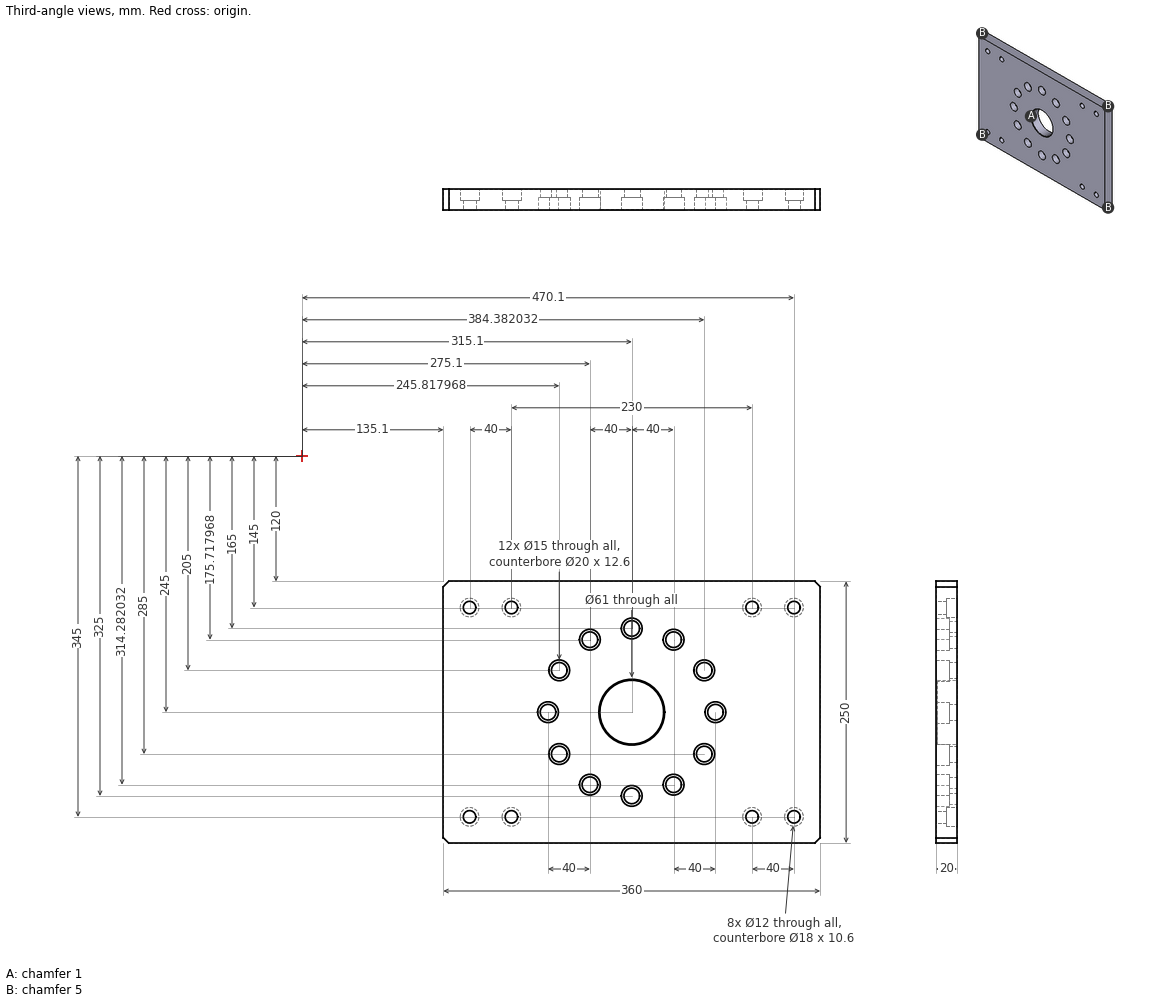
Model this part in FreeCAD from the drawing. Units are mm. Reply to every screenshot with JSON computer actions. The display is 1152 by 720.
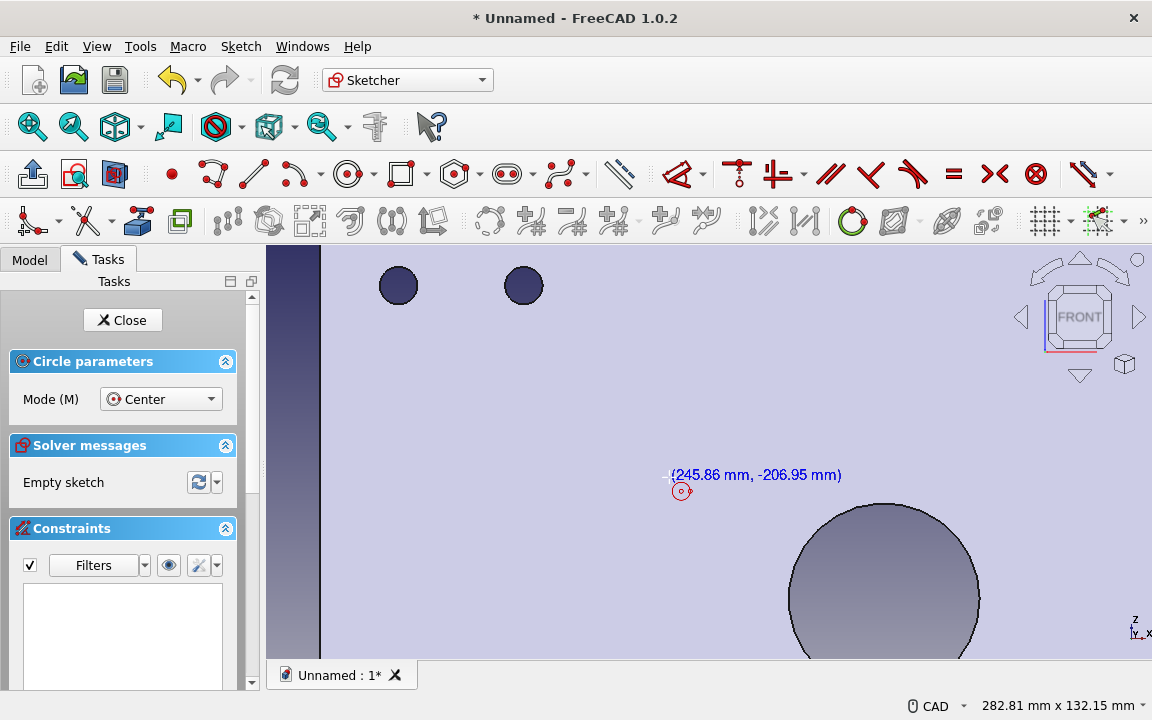
{"action": "scroll", "coordinate": [677, 485], "scroll_direction": "down", "scroll_amount": 7}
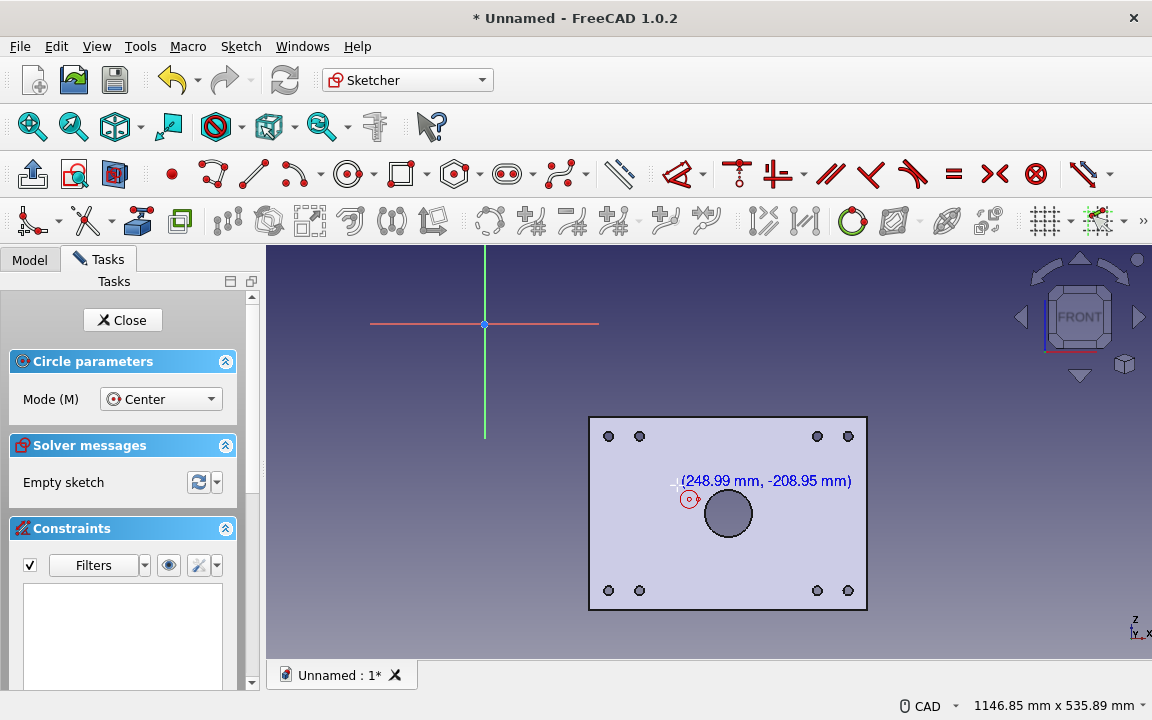
{"action": "left_click", "coordinate": [675, 483]}
{"action": "mouse_move", "coordinate": [679, 479]}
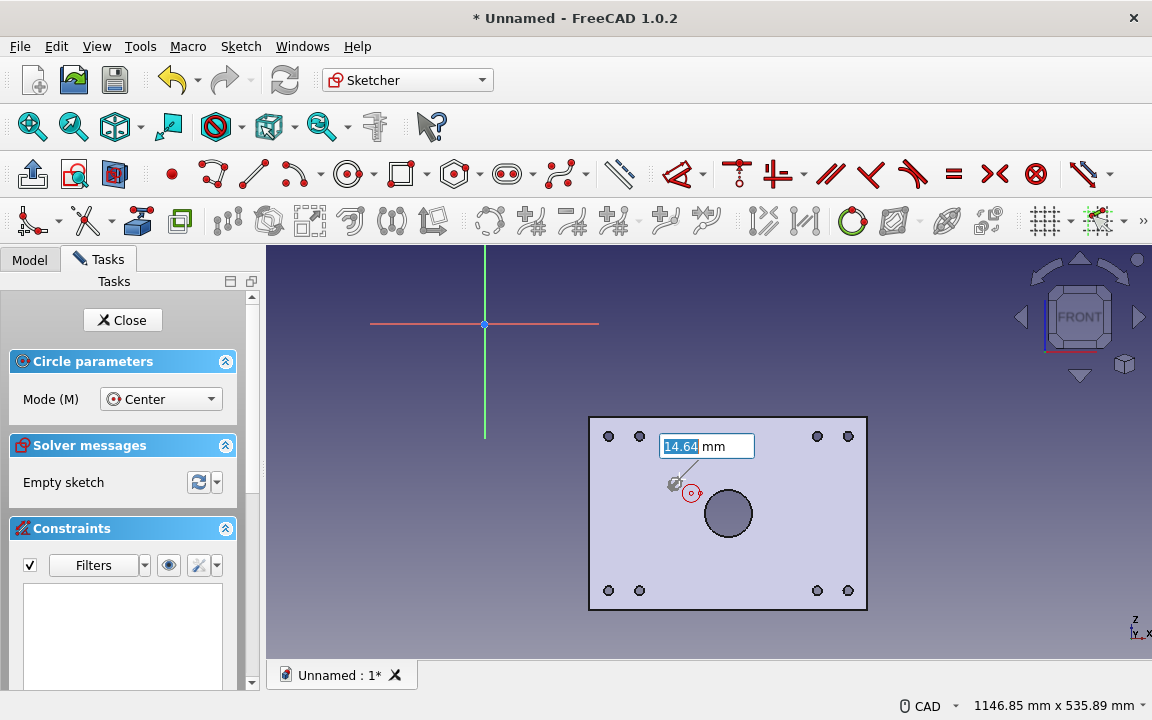
{"action": "type", "text": "15"}
{"action": "key", "text": "Return"}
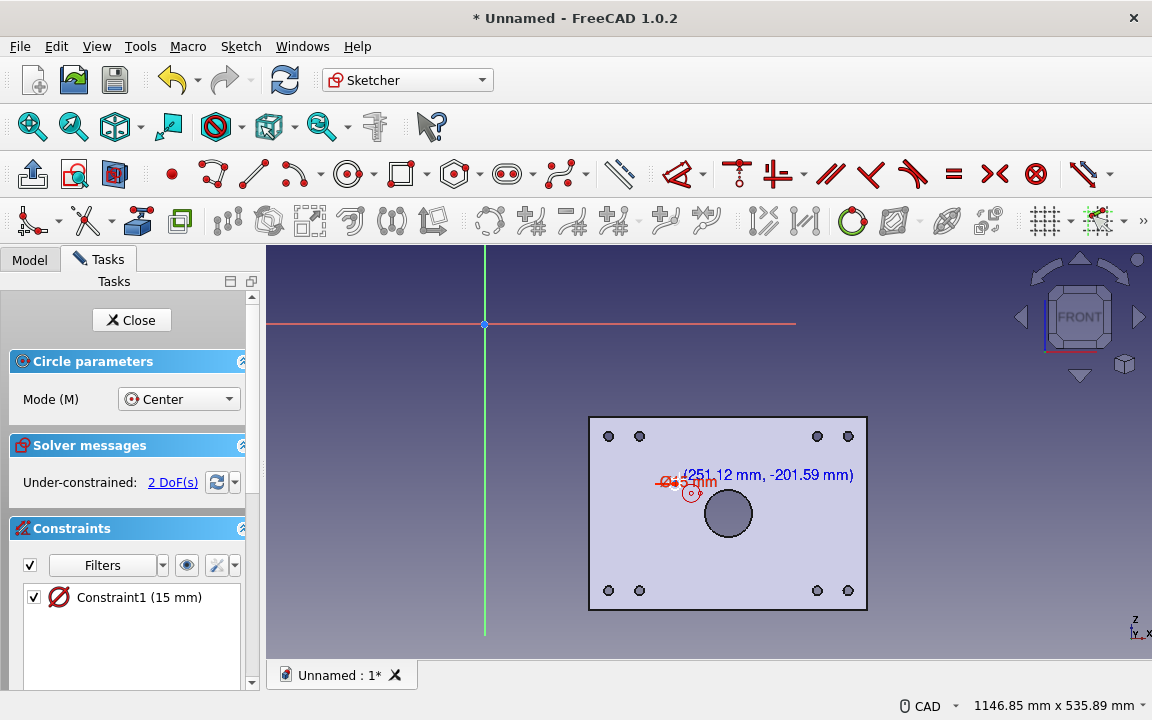
{"action": "scroll", "coordinate": [698, 460], "scroll_direction": "up", "scroll_amount": 7}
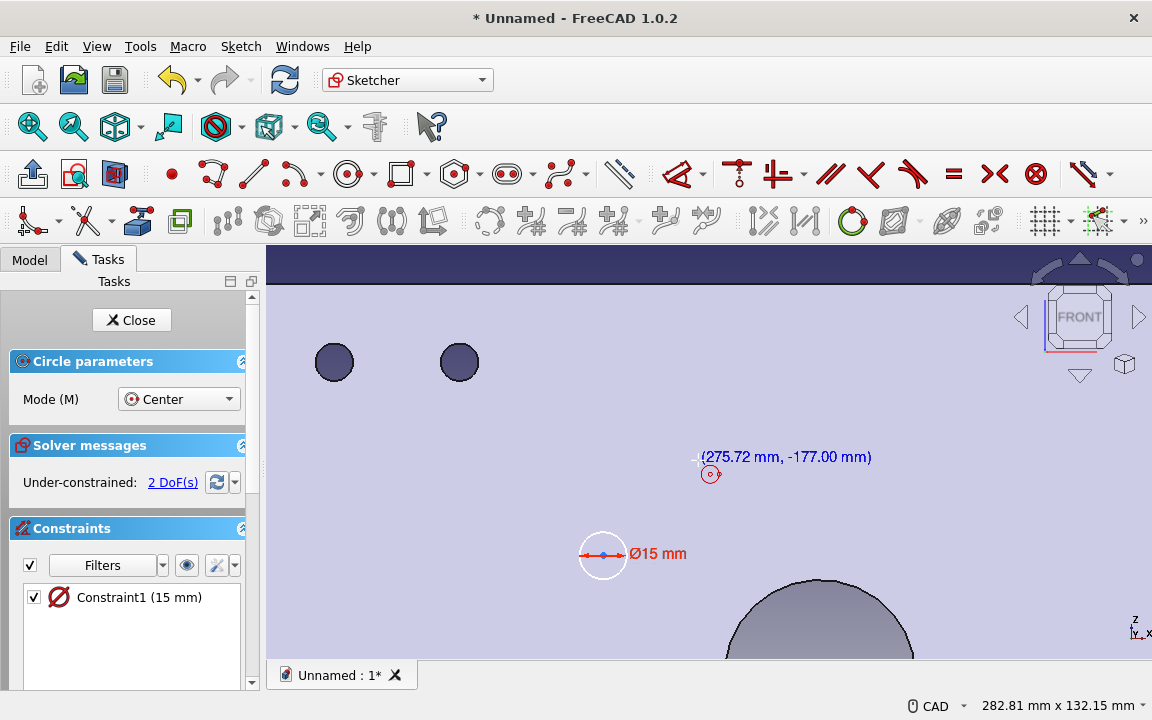
{"action": "scroll", "coordinate": [698, 460], "scroll_direction": "down", "scroll_amount": 7}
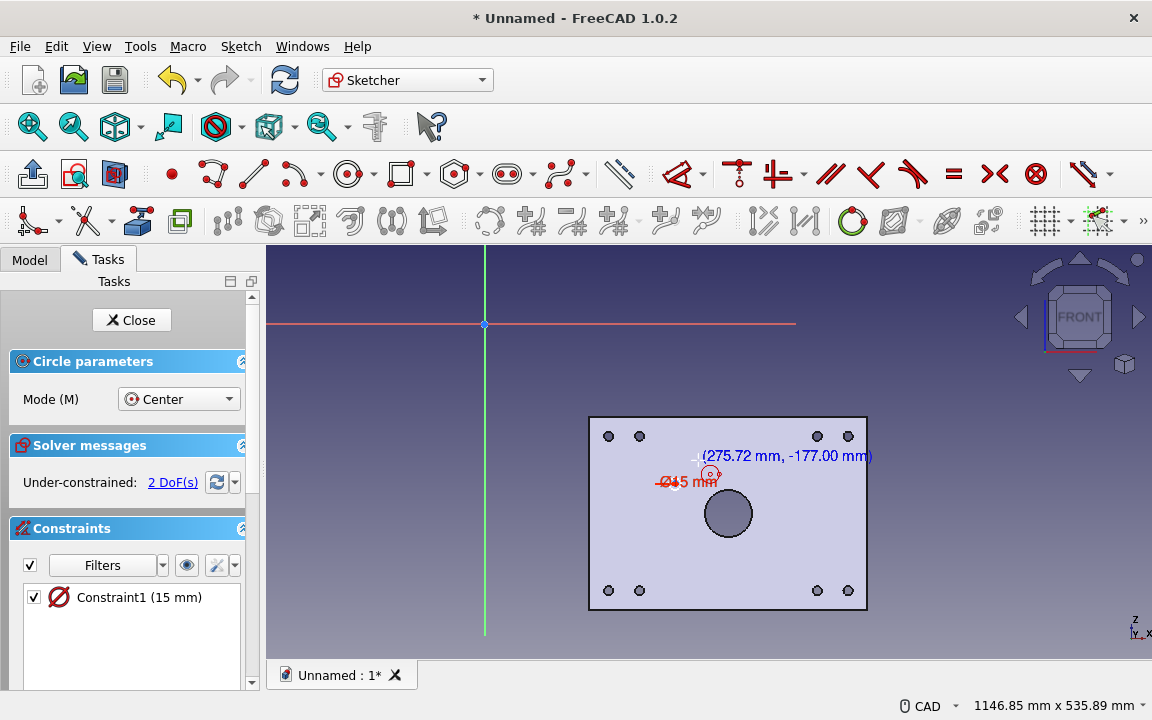
{"action": "left_click", "coordinate": [698, 460]}
{"action": "mouse_move", "coordinate": [702, 456]}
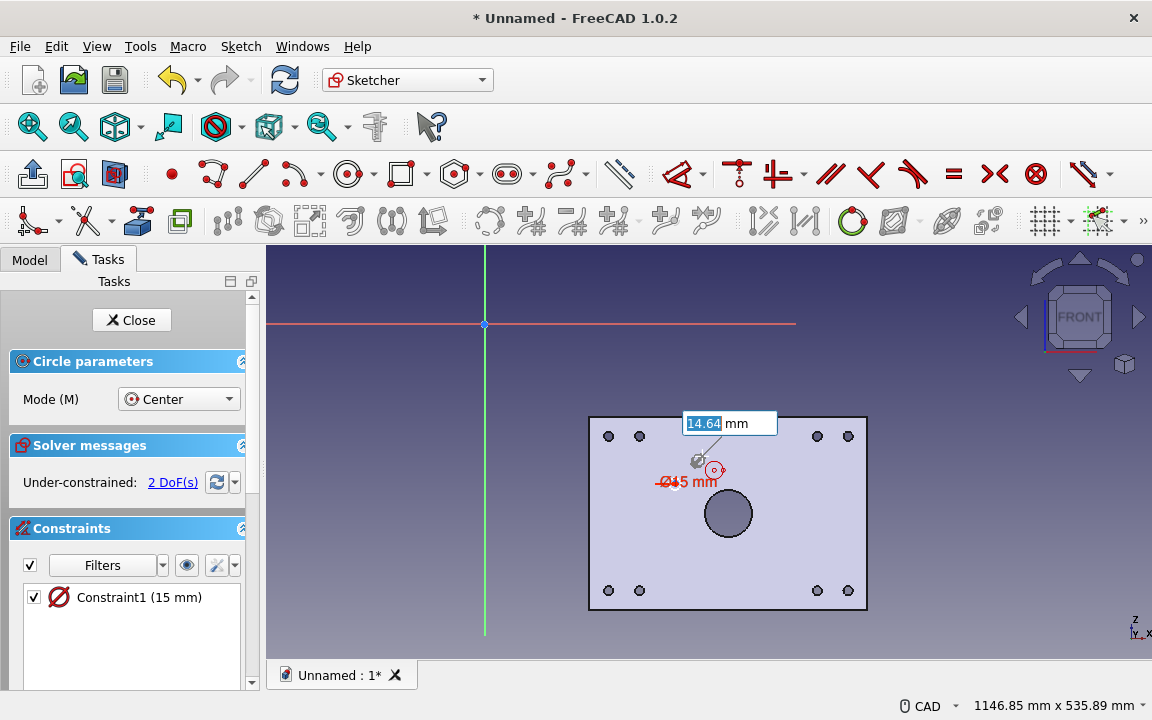
{"action": "type", "text": "15"}
{"action": "key", "text": "Return"}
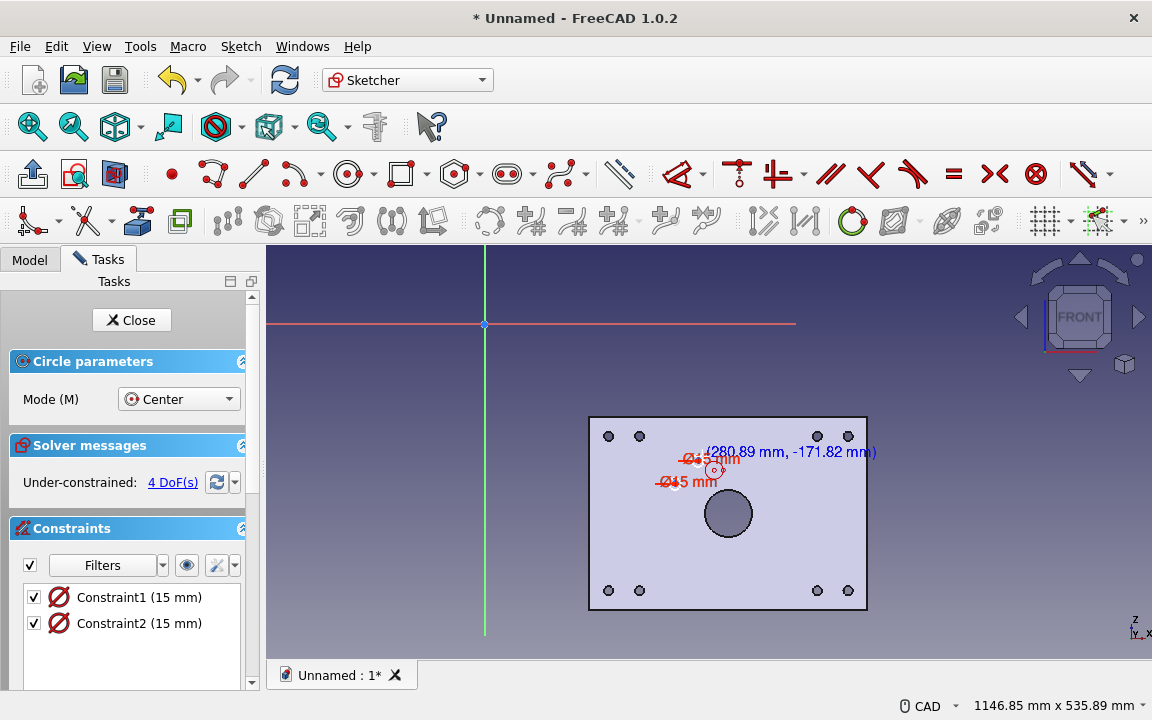
{"action": "scroll", "coordinate": [728, 452], "scroll_direction": "up", "scroll_amount": 7}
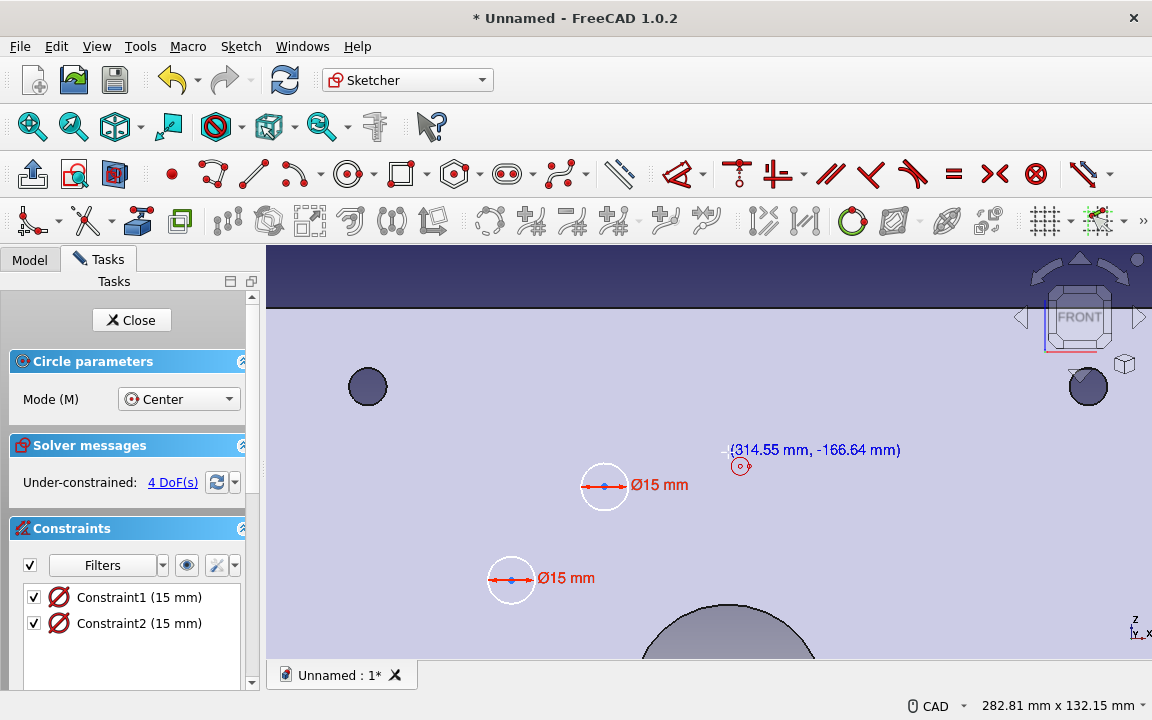
{"action": "scroll", "coordinate": [729, 452], "scroll_direction": "down", "scroll_amount": 7}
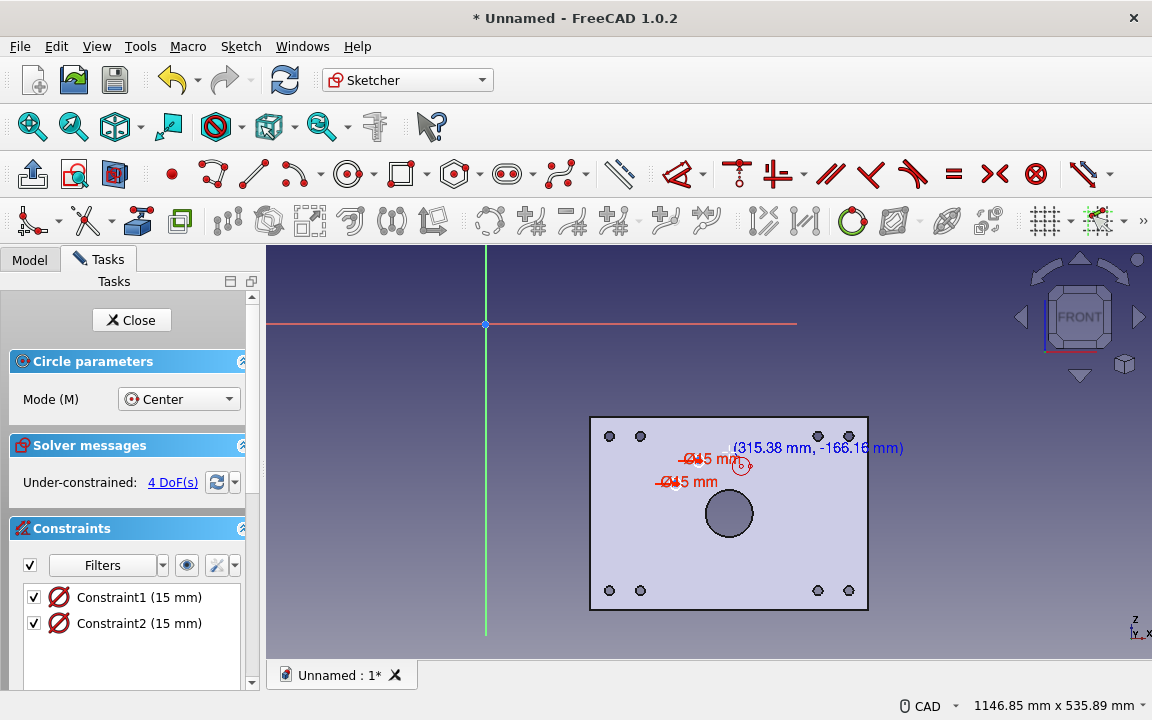
{"action": "left_click", "coordinate": [729, 452]}
{"action": "mouse_move", "coordinate": [733, 448]}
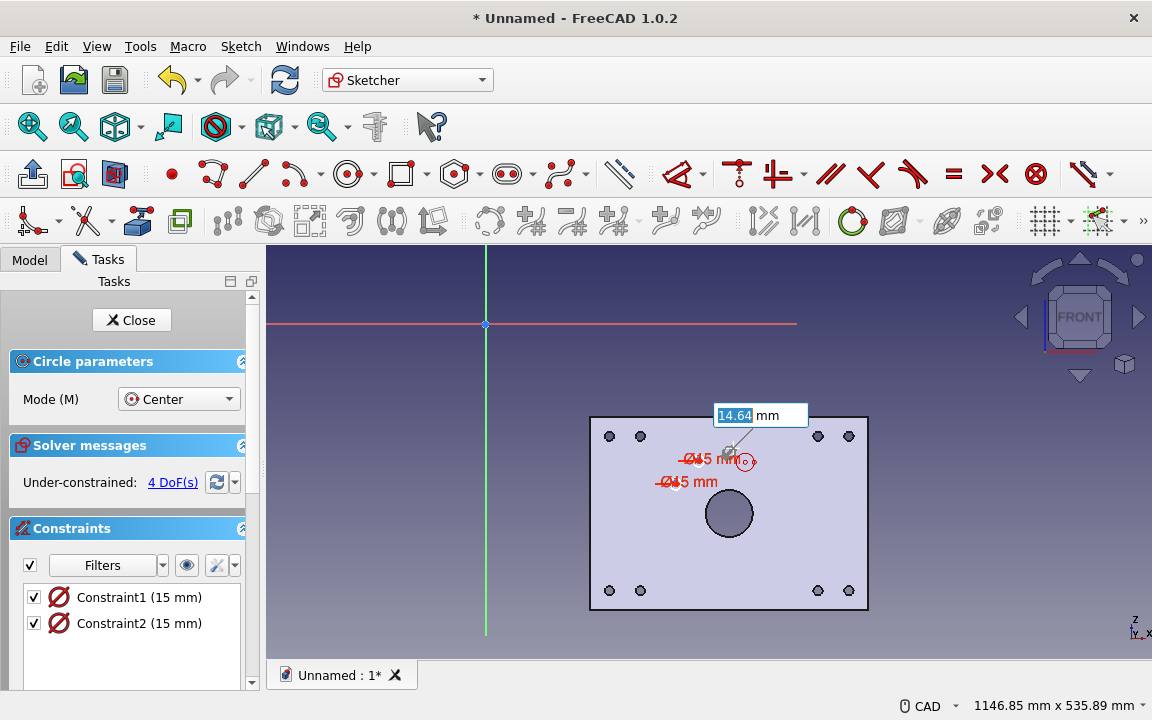
{"action": "type", "text": "15"}
{"action": "key", "text": "Return"}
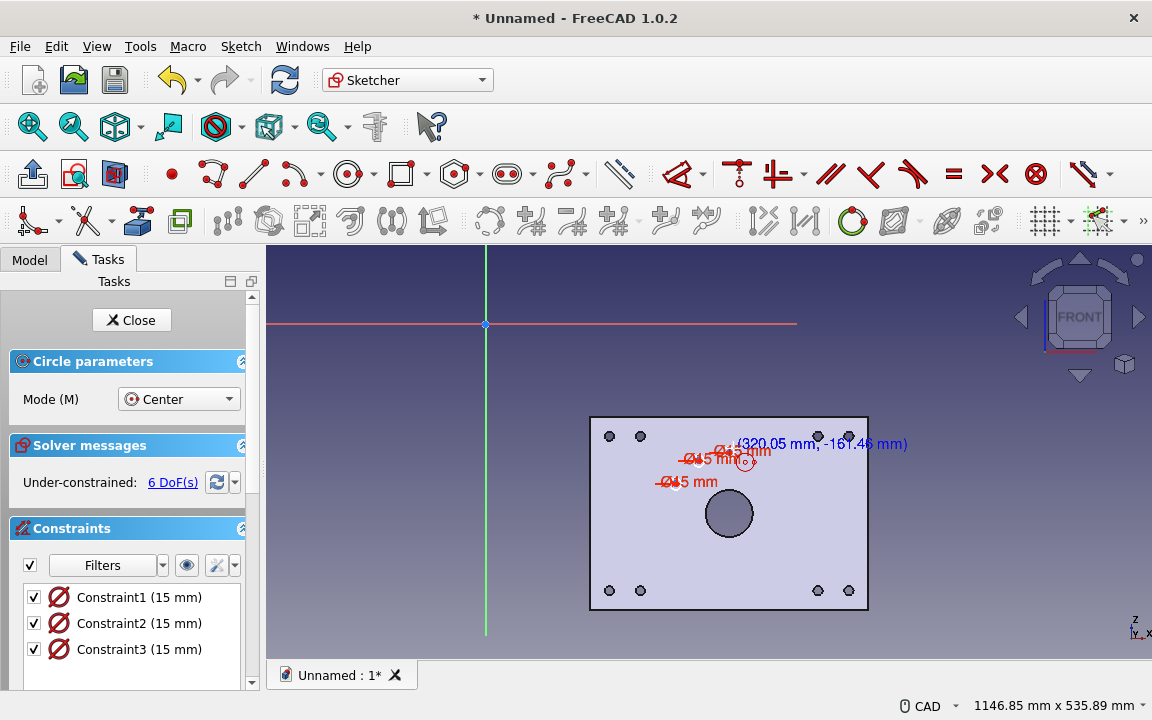
{"action": "scroll", "coordinate": [760, 460], "scroll_direction": "up", "scroll_amount": 7}